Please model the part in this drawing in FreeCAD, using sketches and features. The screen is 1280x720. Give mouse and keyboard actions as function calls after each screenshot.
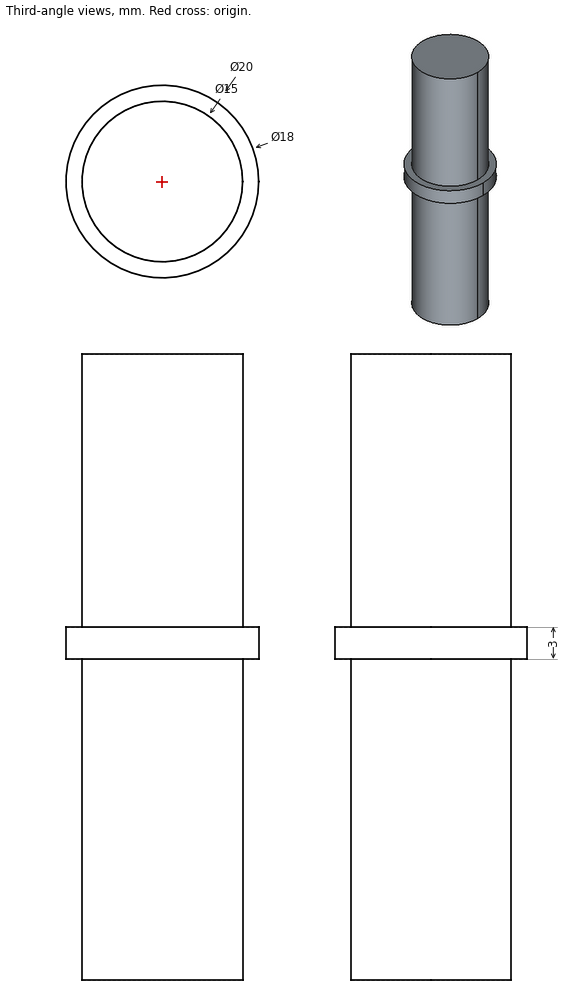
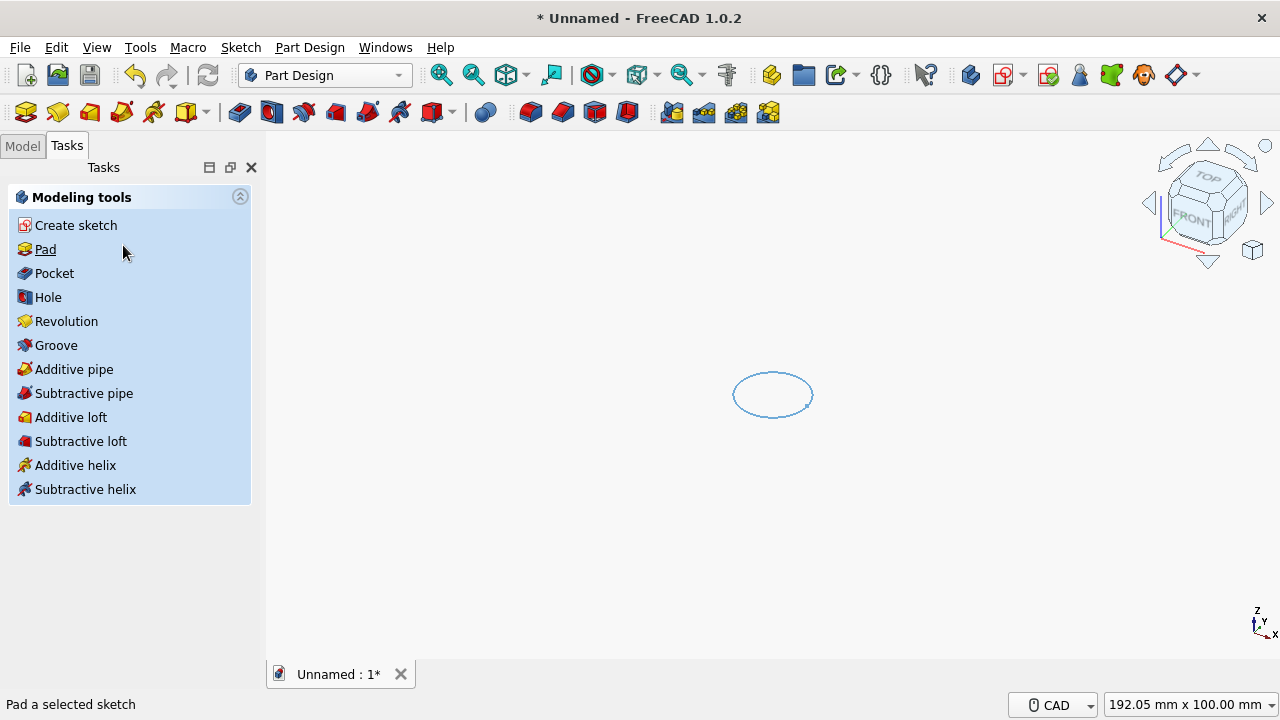
click(26, 112)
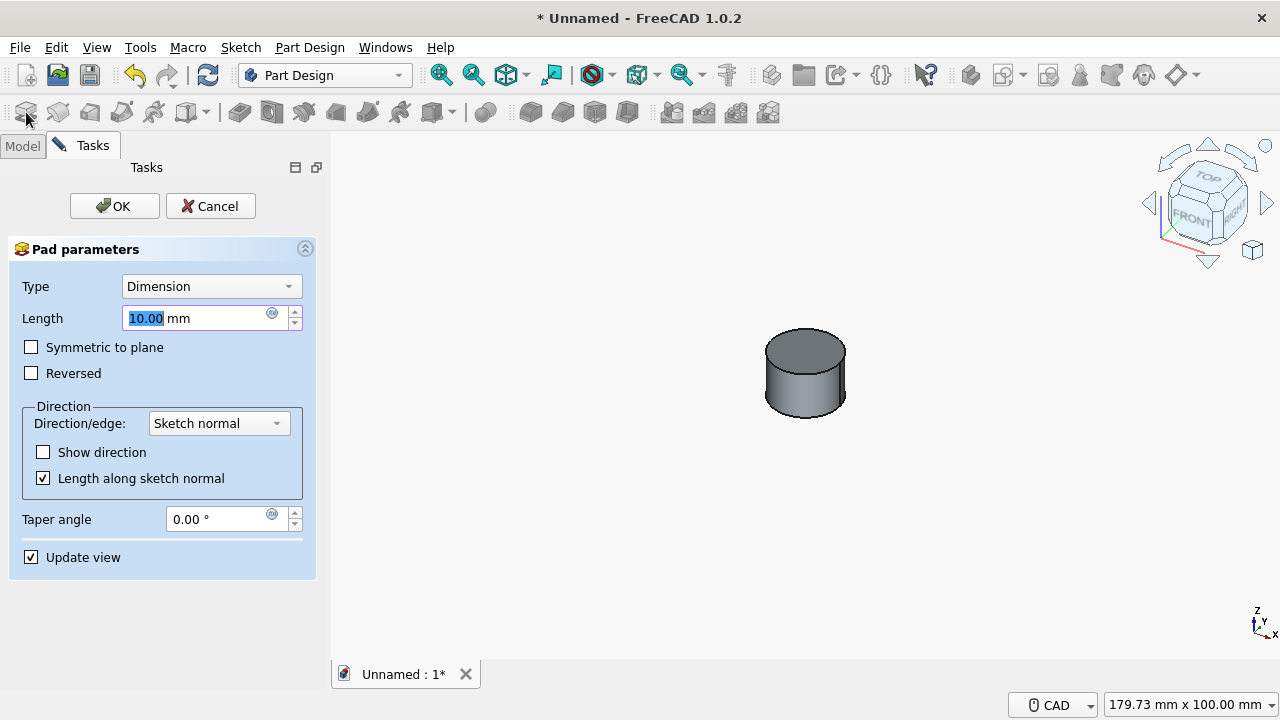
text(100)
key(Tab)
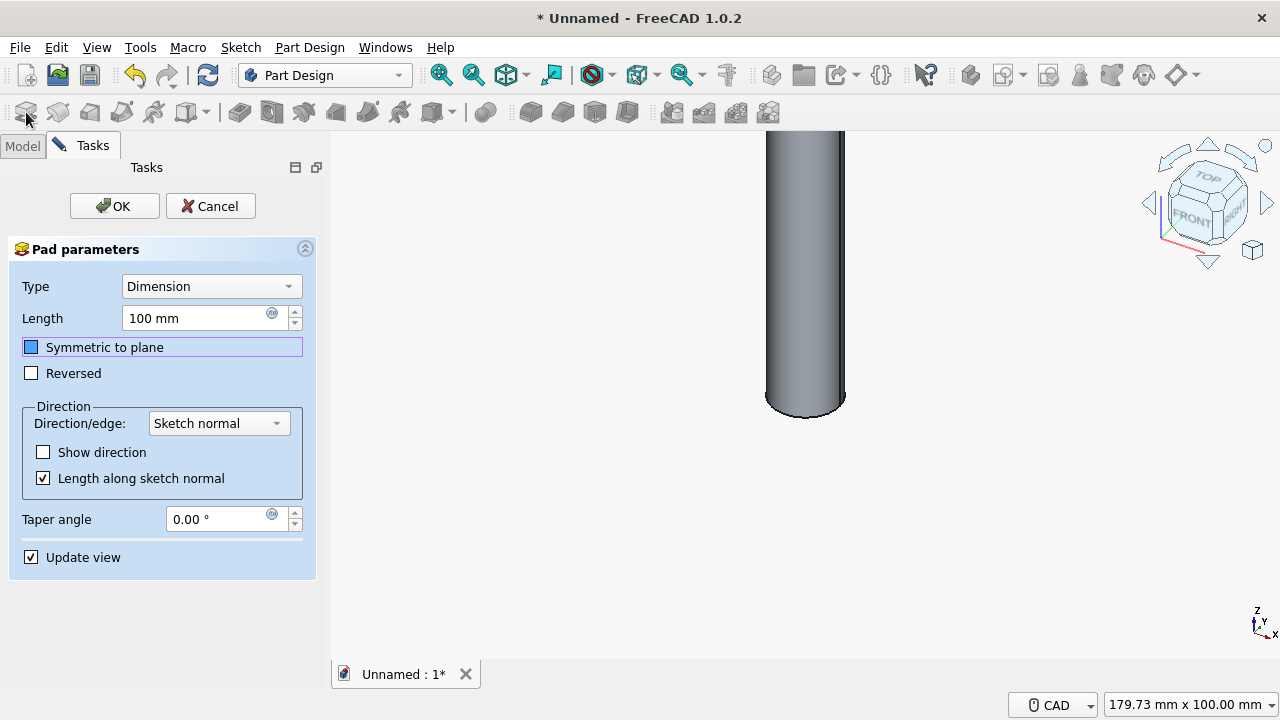
click(115, 206)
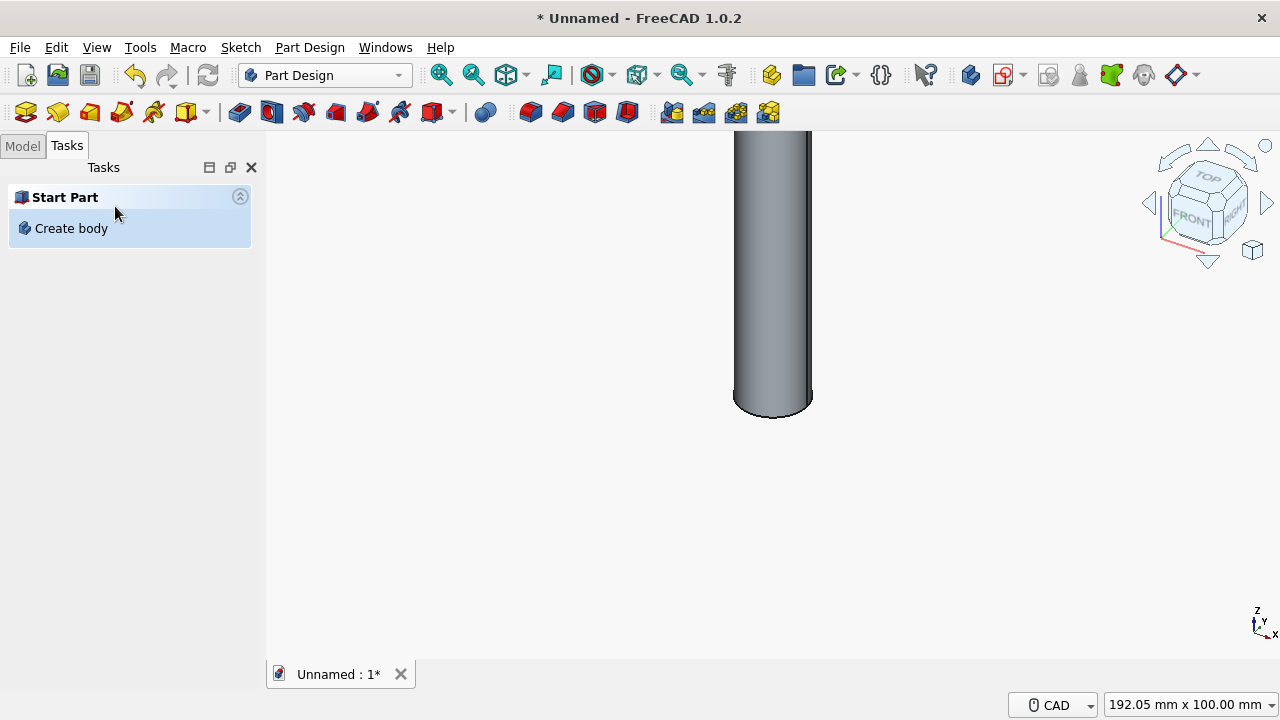
click(442, 76)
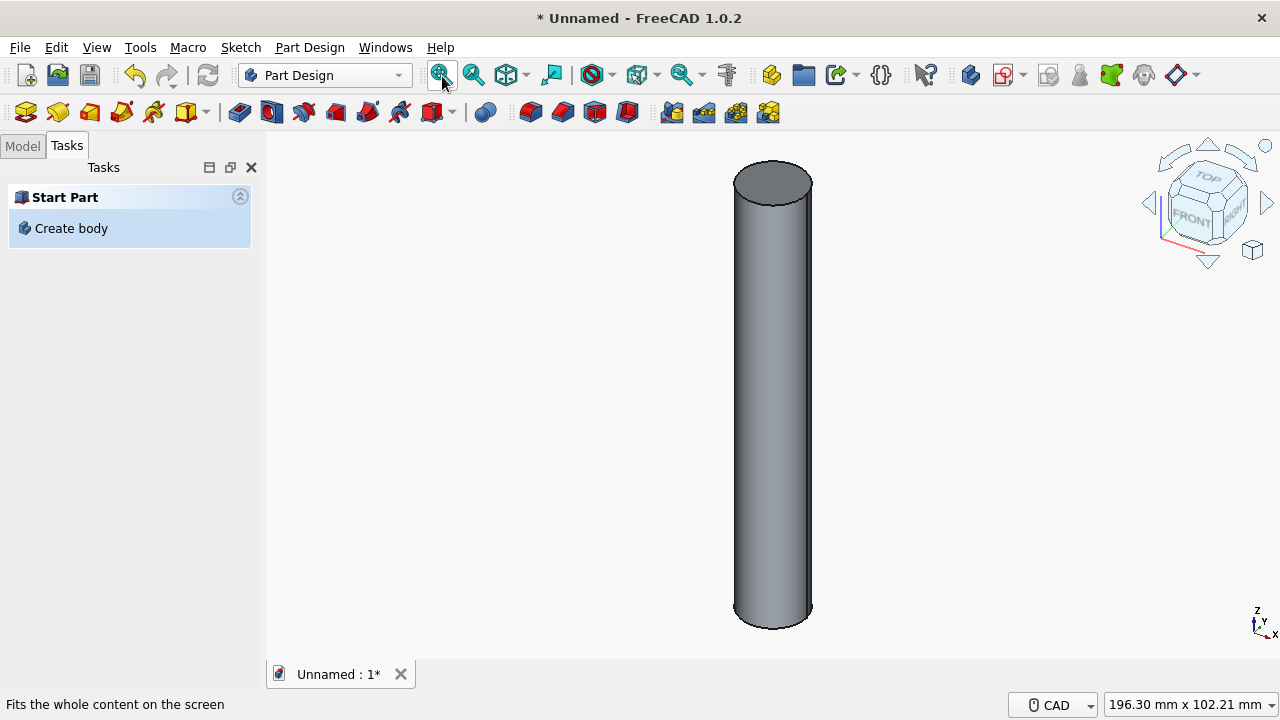
click(23, 145)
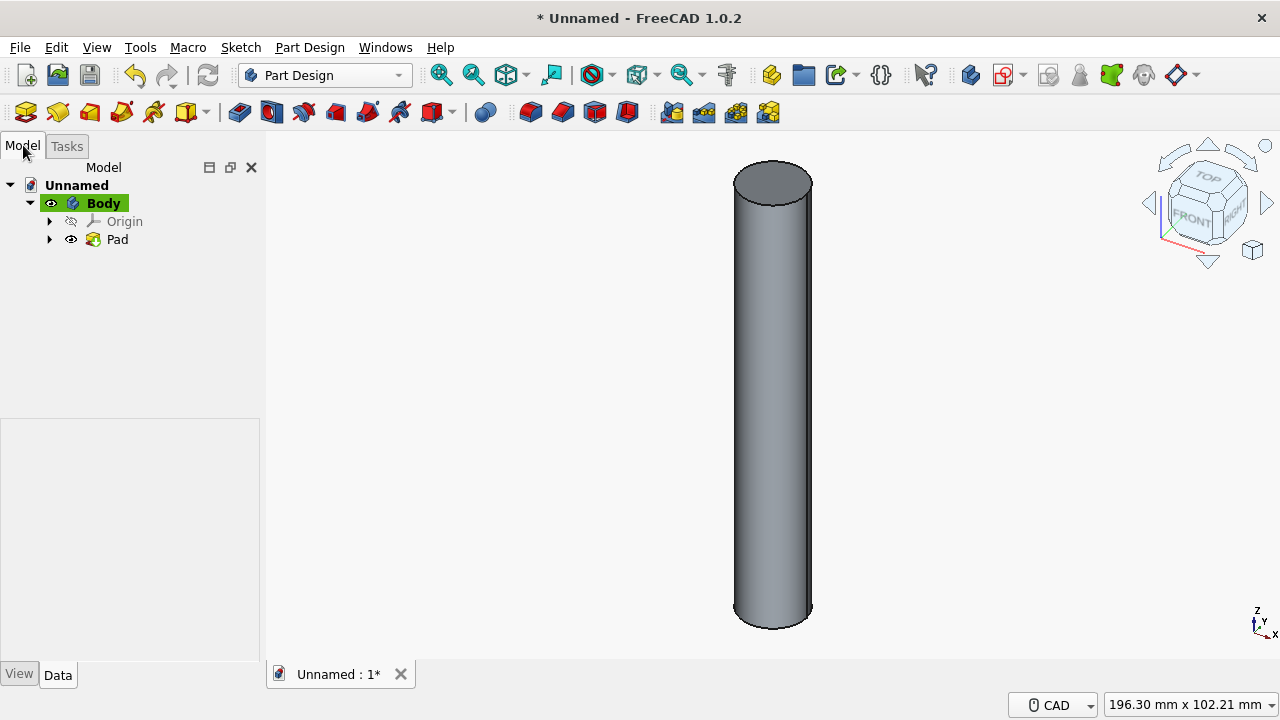
click(50, 221)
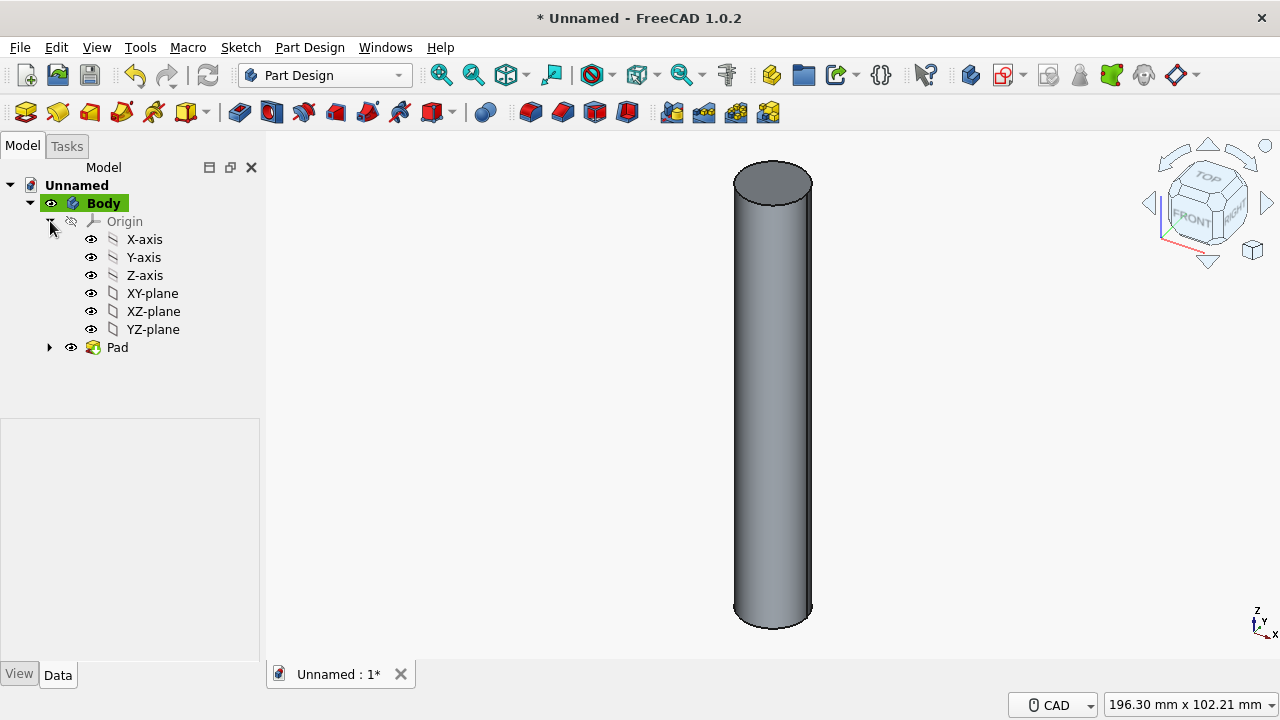
click(136, 293)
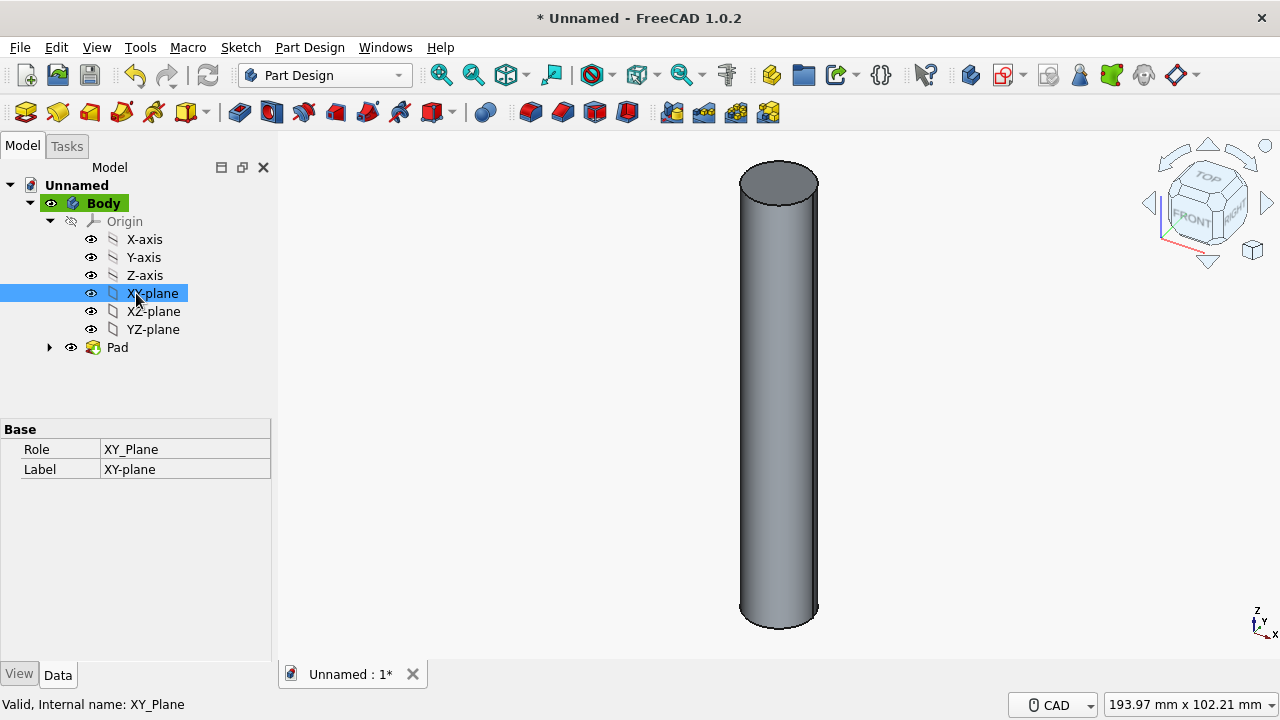
click(1176, 76)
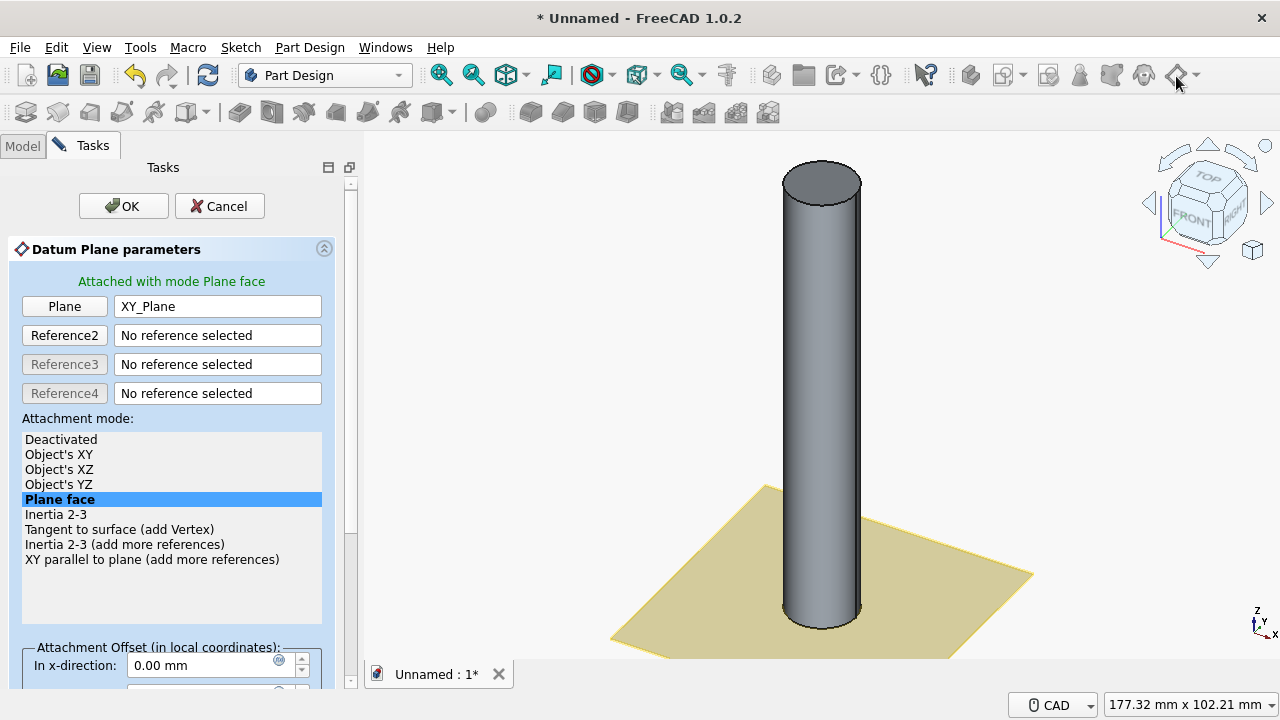
scroll(351, 432, down, 2)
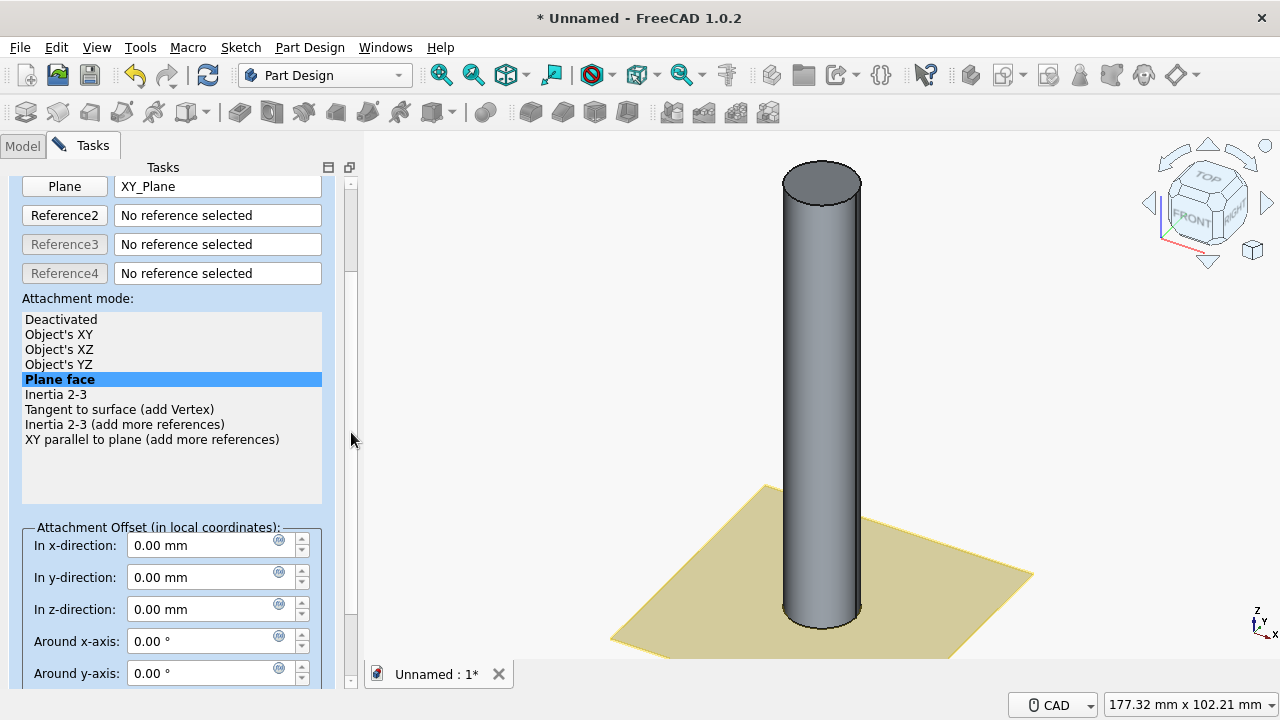
triple_click(210, 609)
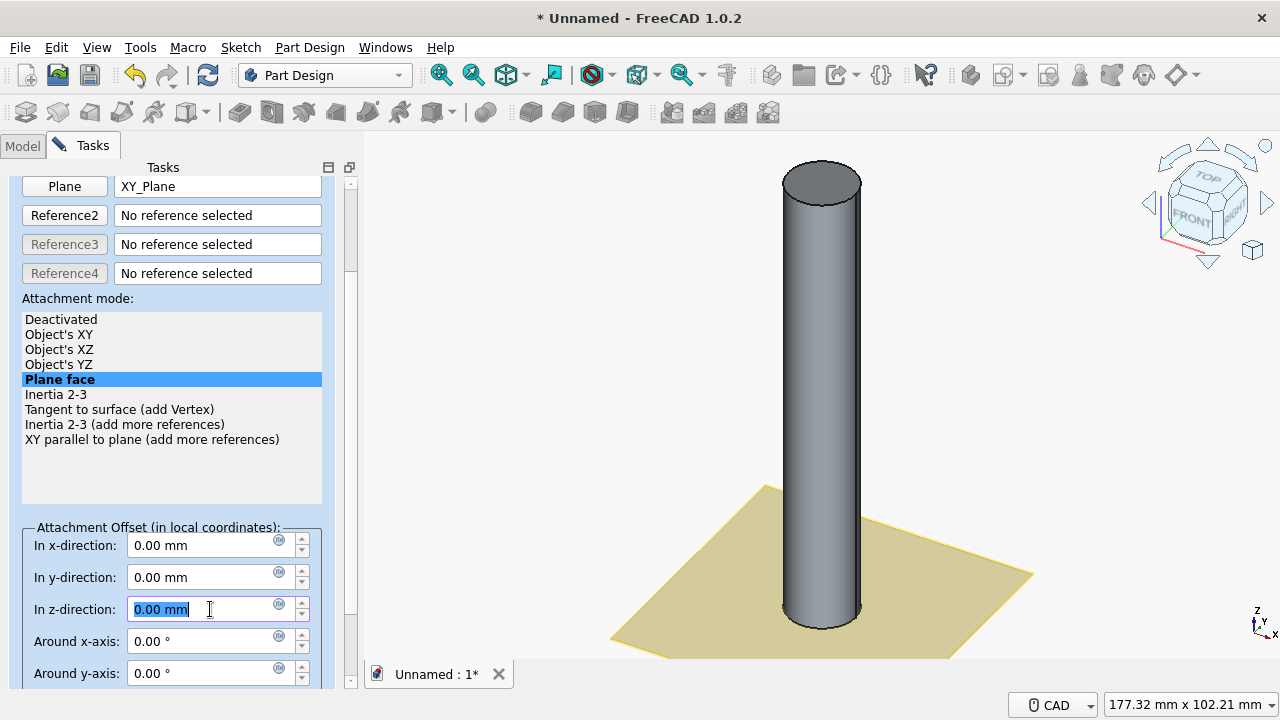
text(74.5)
key(Tab)